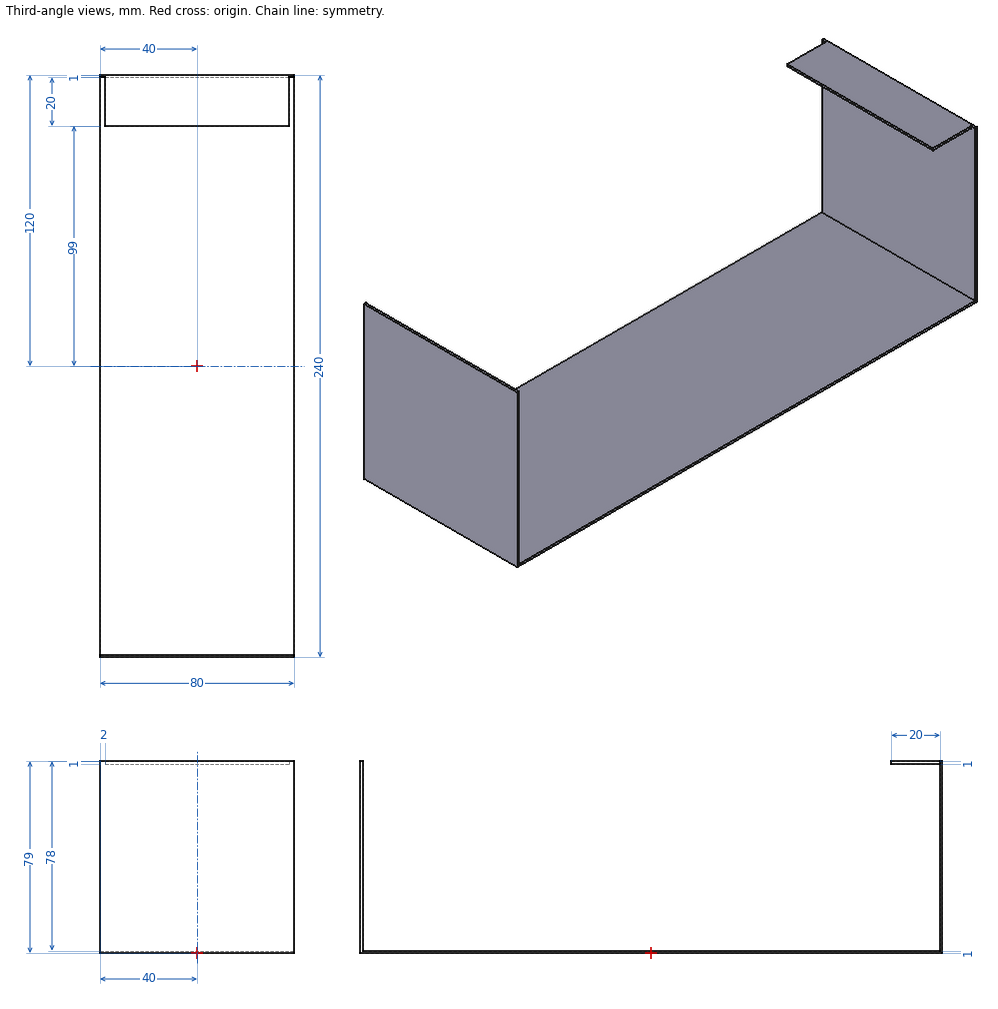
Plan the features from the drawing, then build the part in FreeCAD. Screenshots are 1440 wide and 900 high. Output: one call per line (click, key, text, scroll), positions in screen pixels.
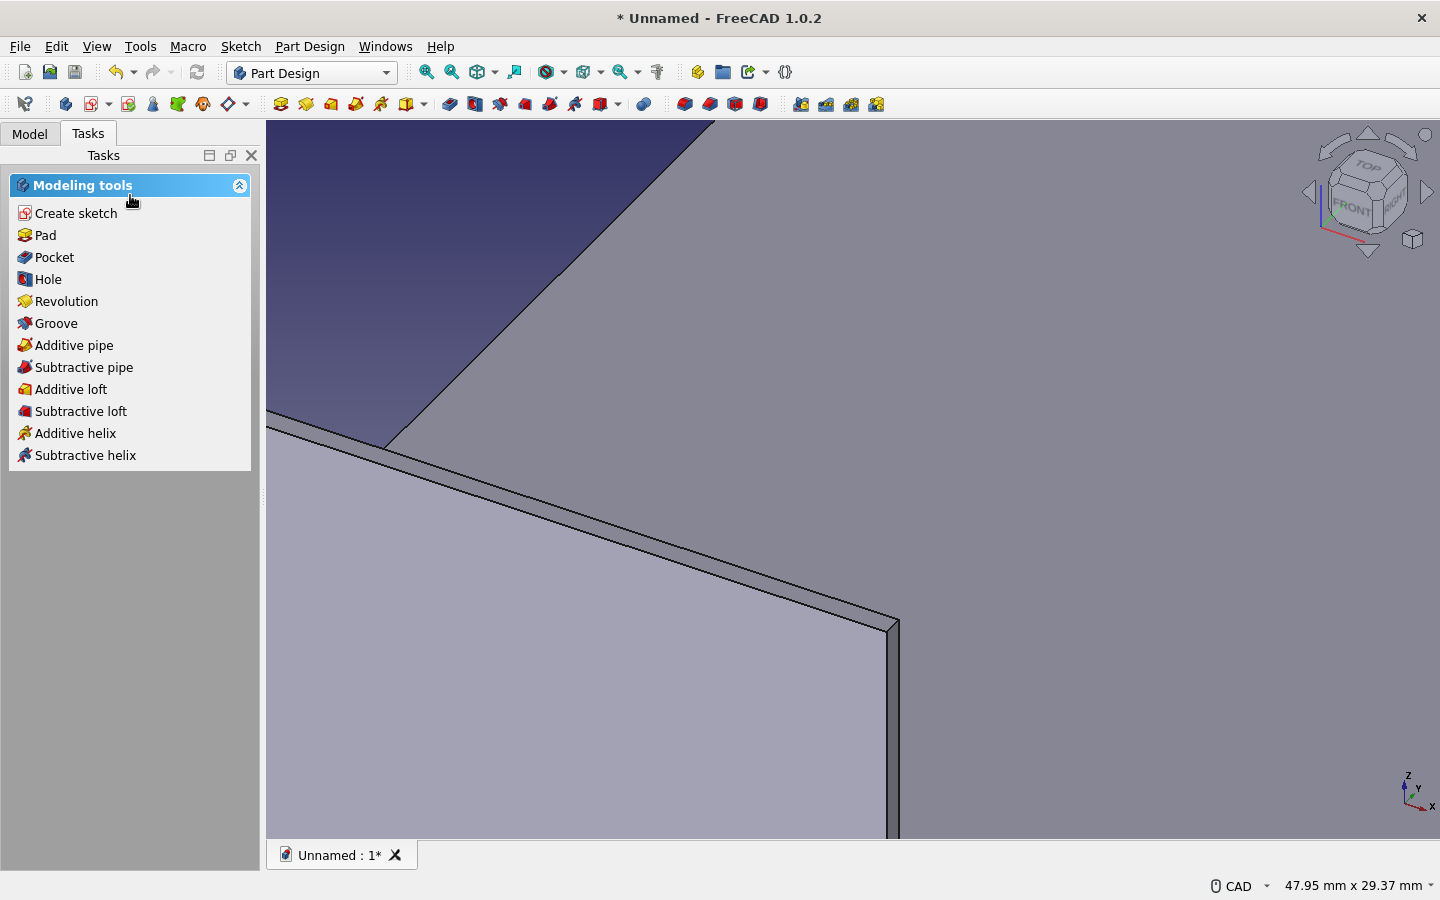
click(281, 104)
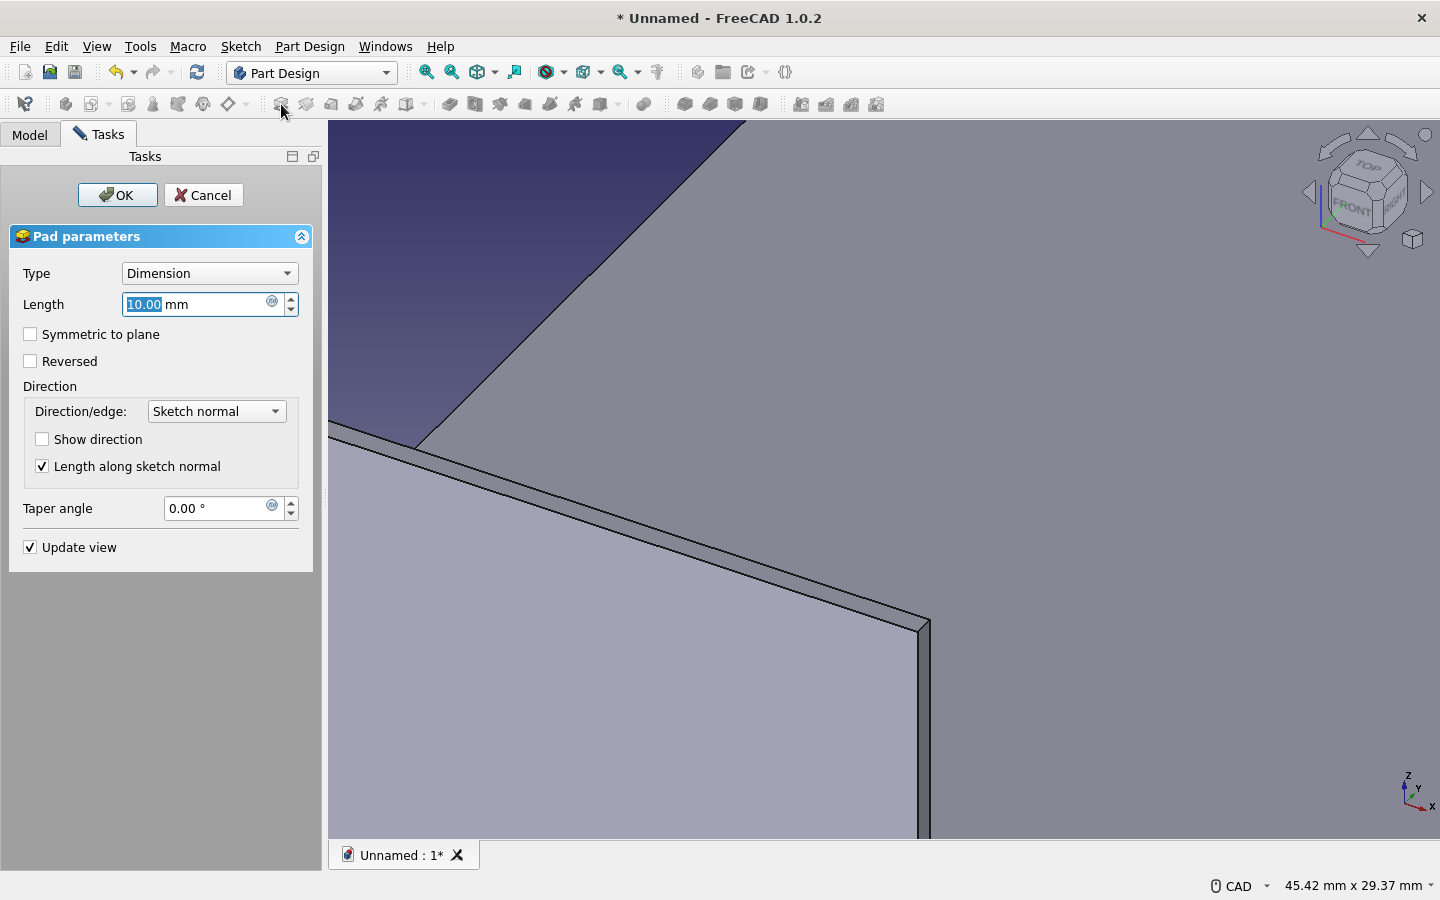
text(1)
key(Tab)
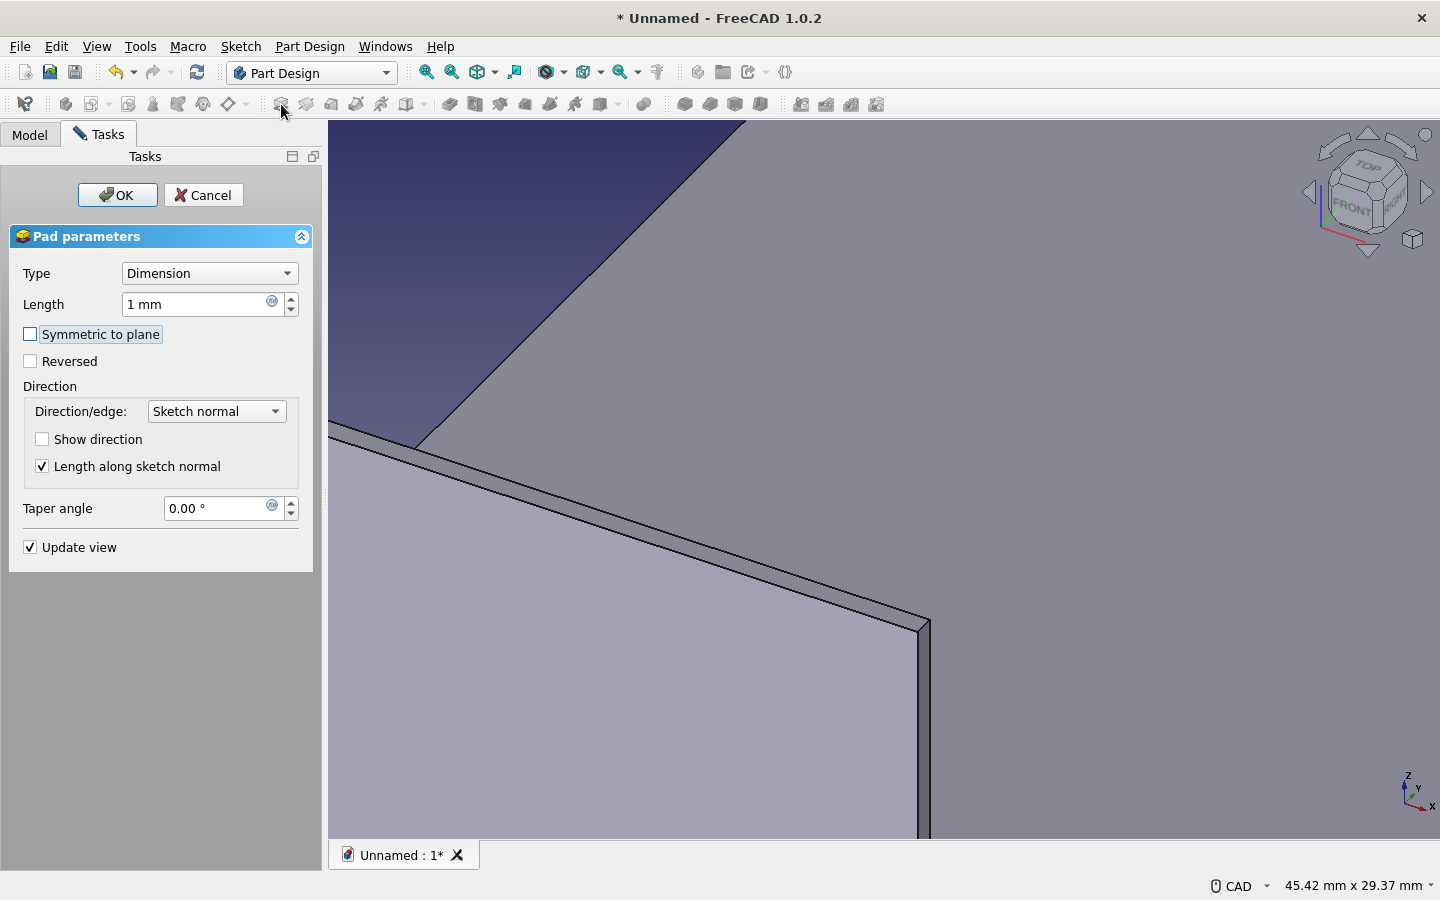
click(31, 361)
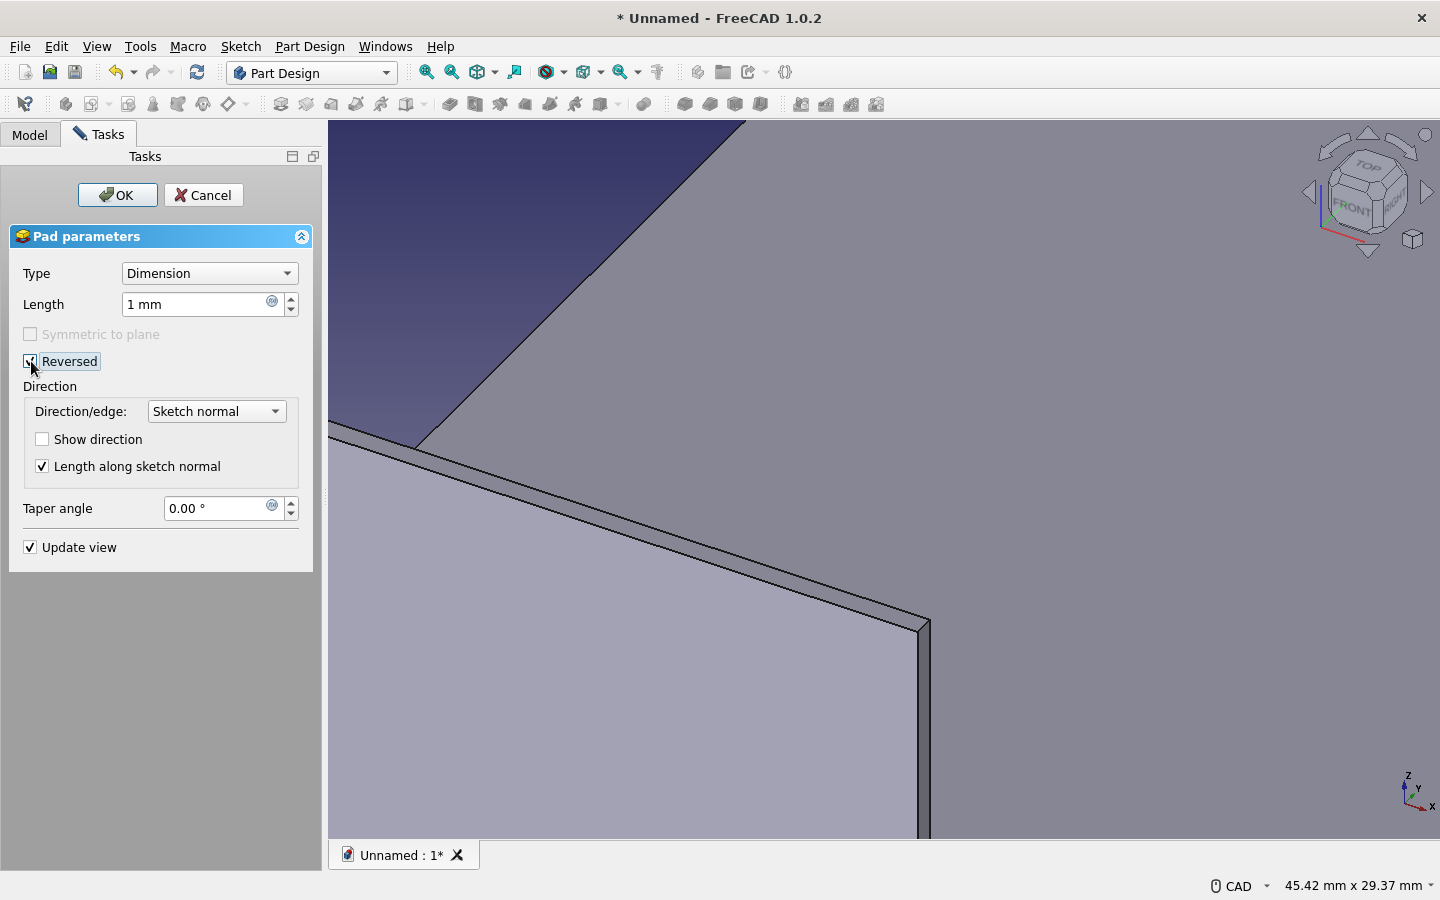
click(118, 195)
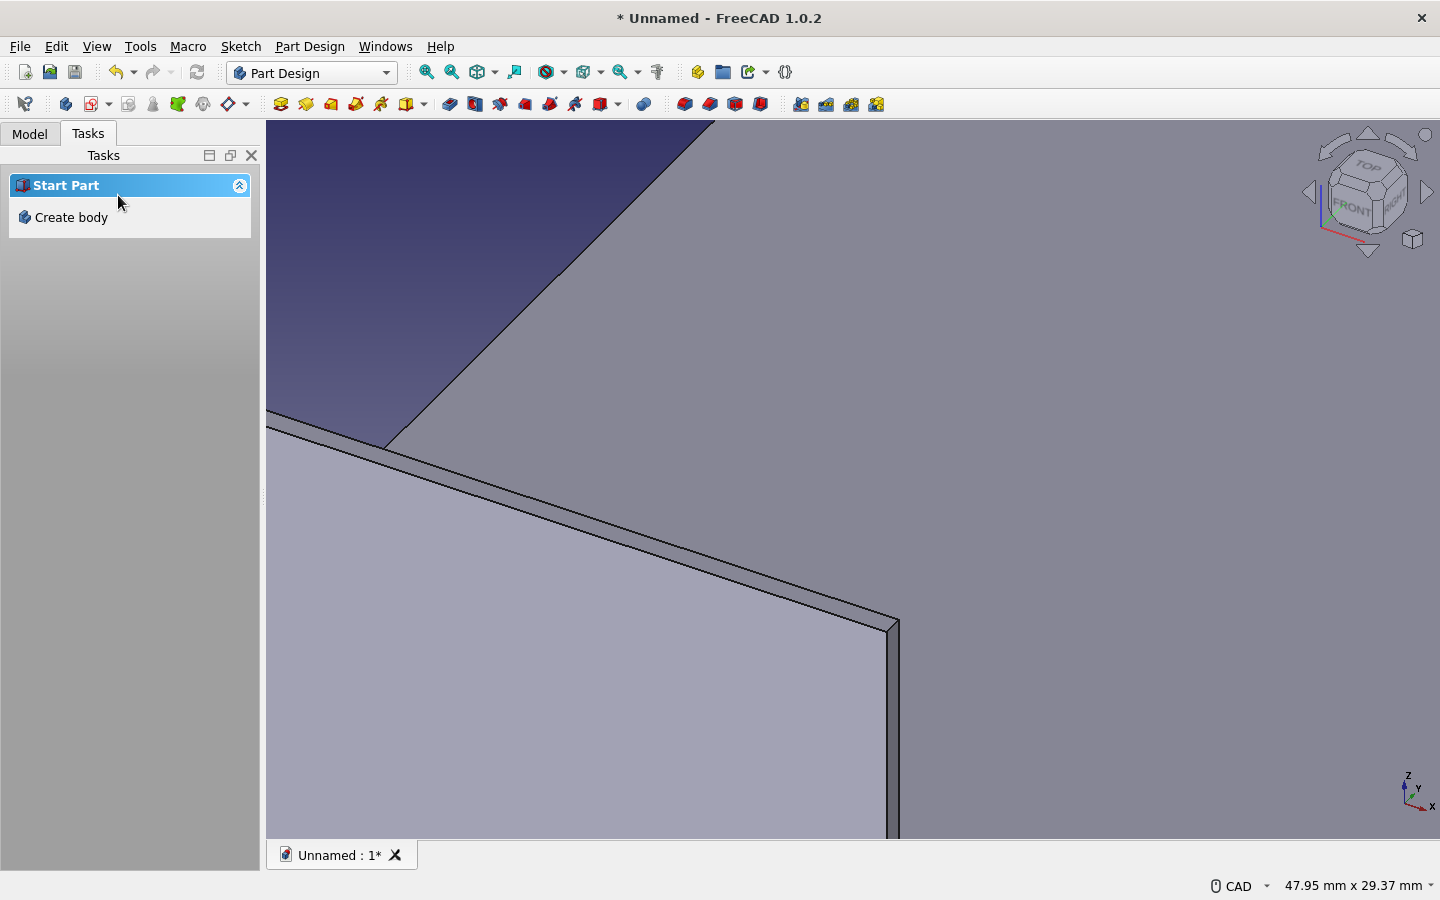
click(427, 72)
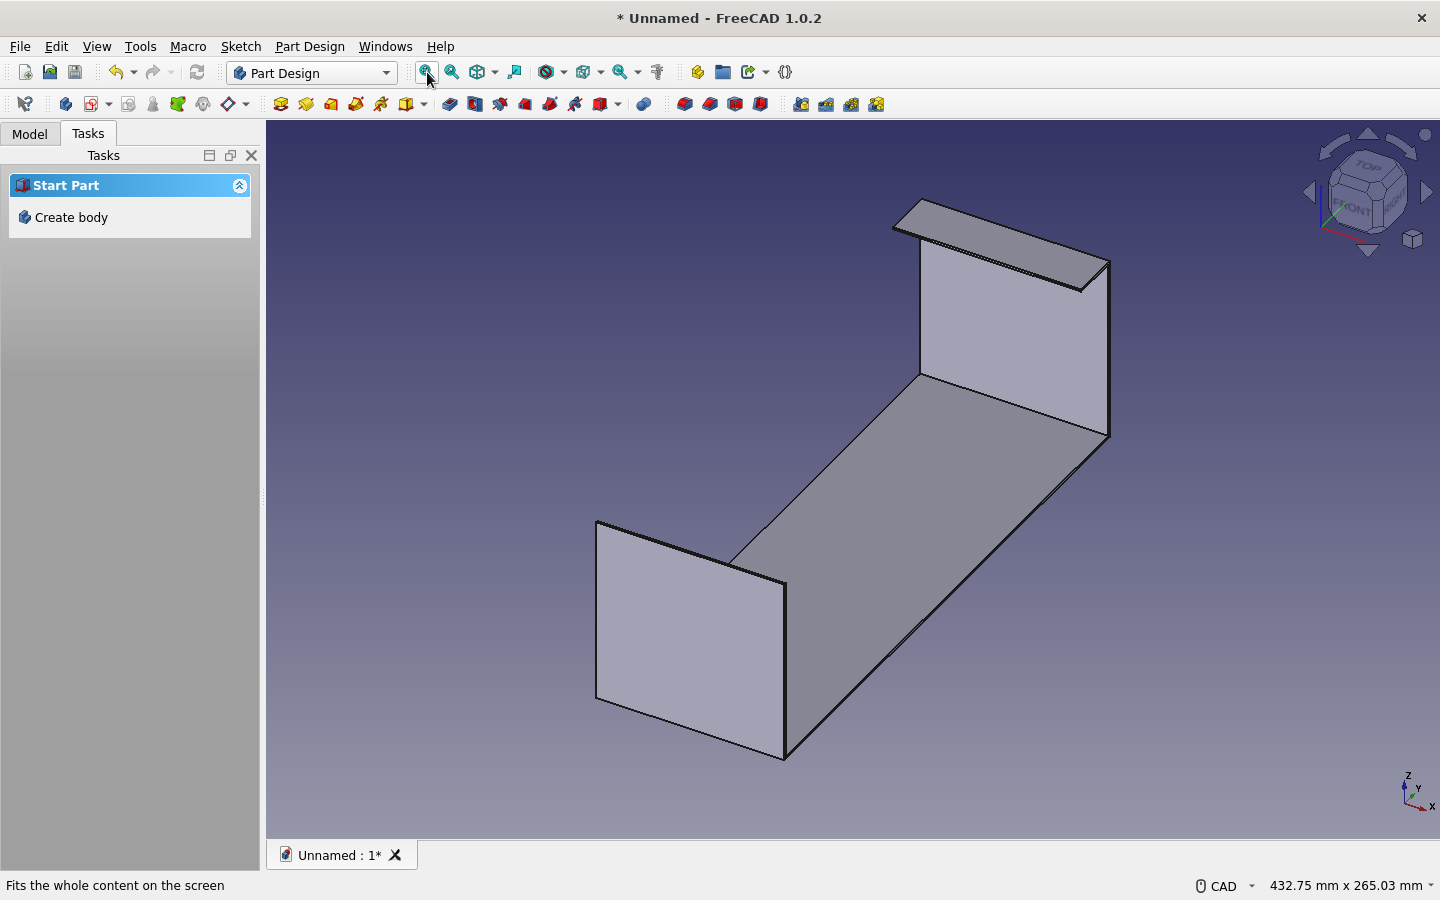
click(30, 134)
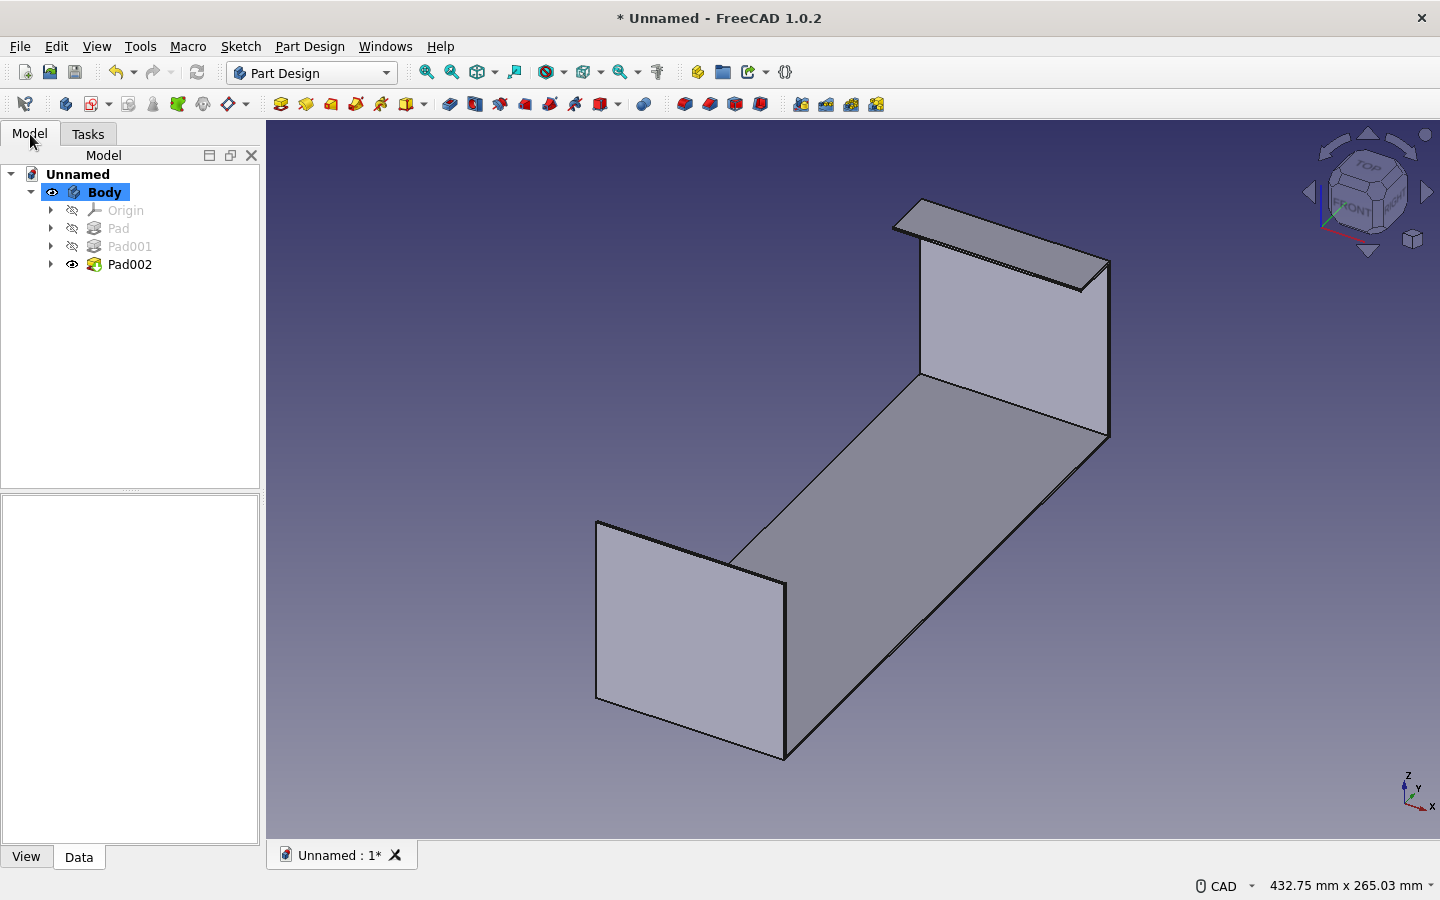
click(51, 210)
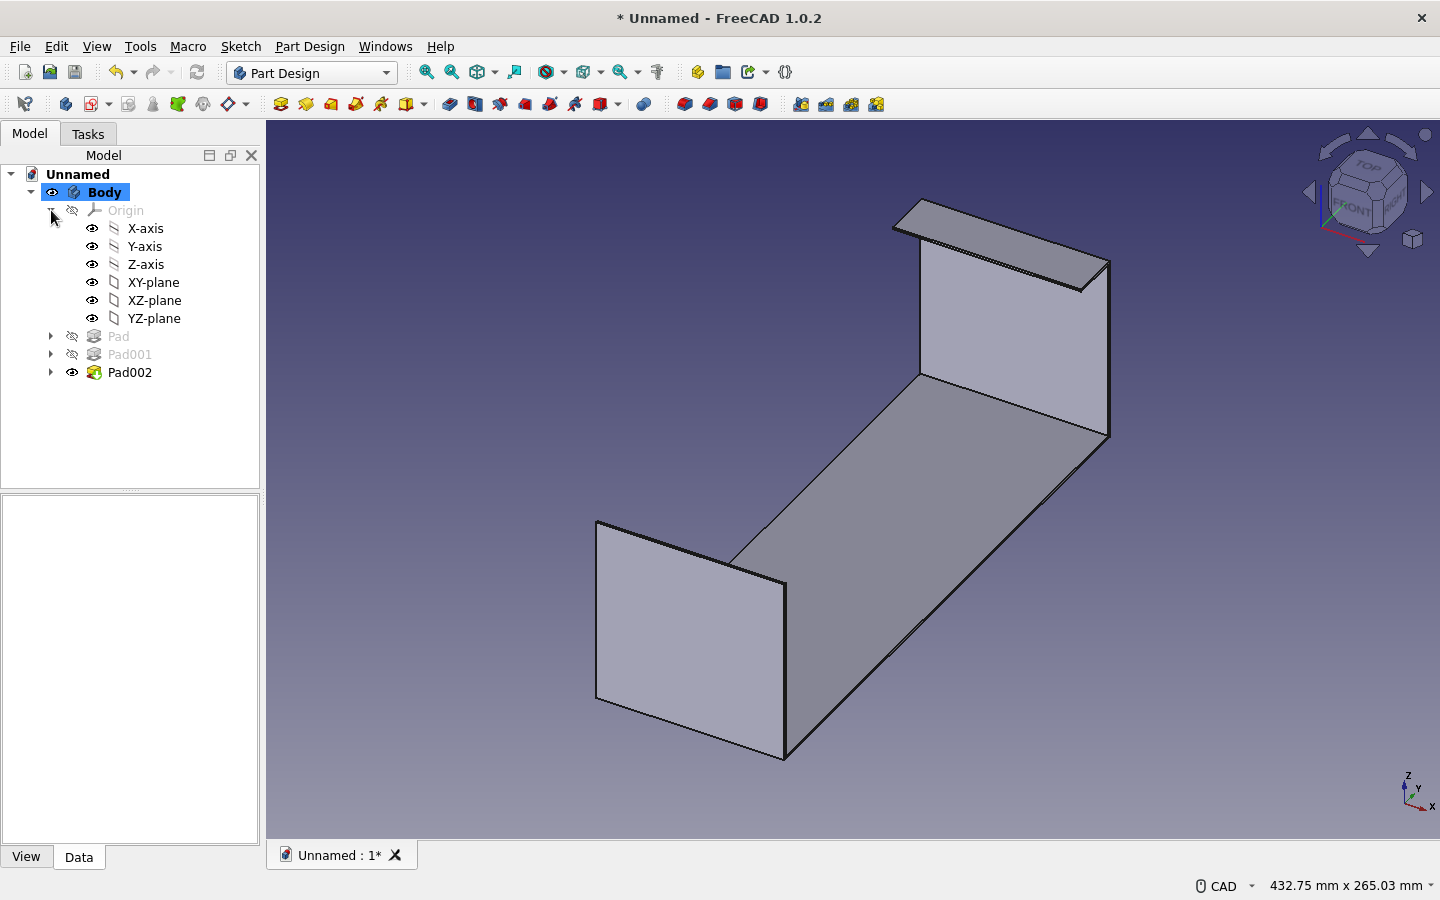
click(137, 300)